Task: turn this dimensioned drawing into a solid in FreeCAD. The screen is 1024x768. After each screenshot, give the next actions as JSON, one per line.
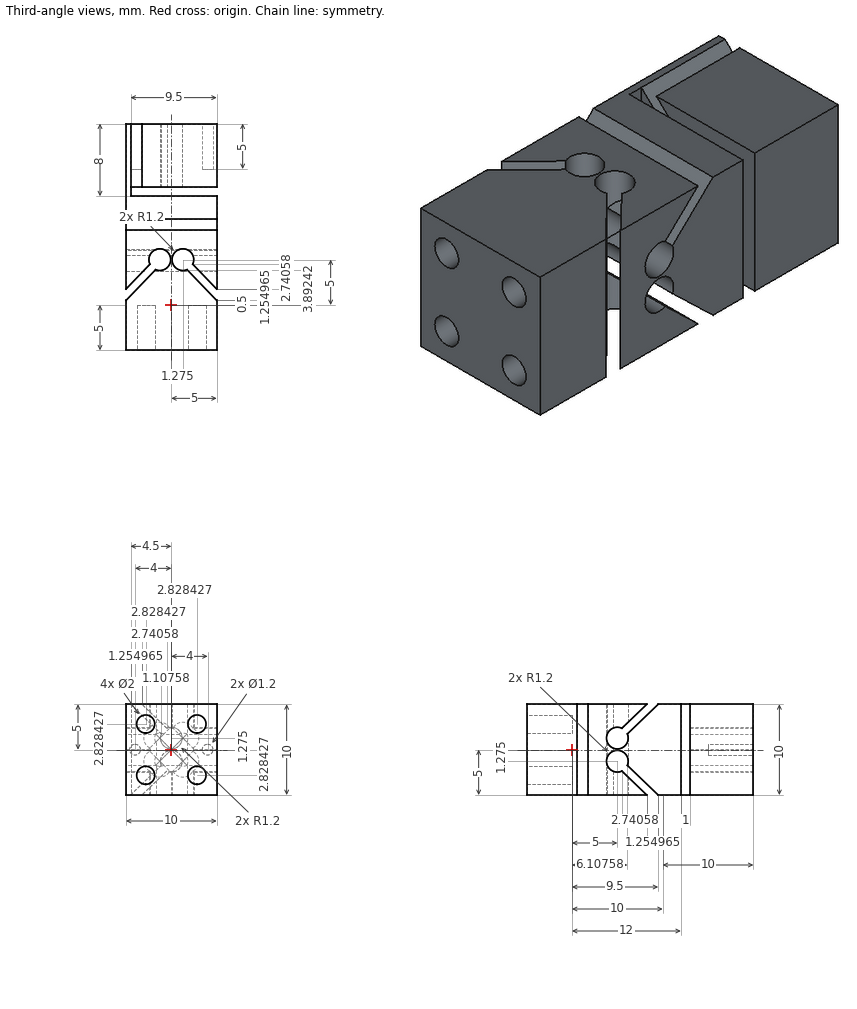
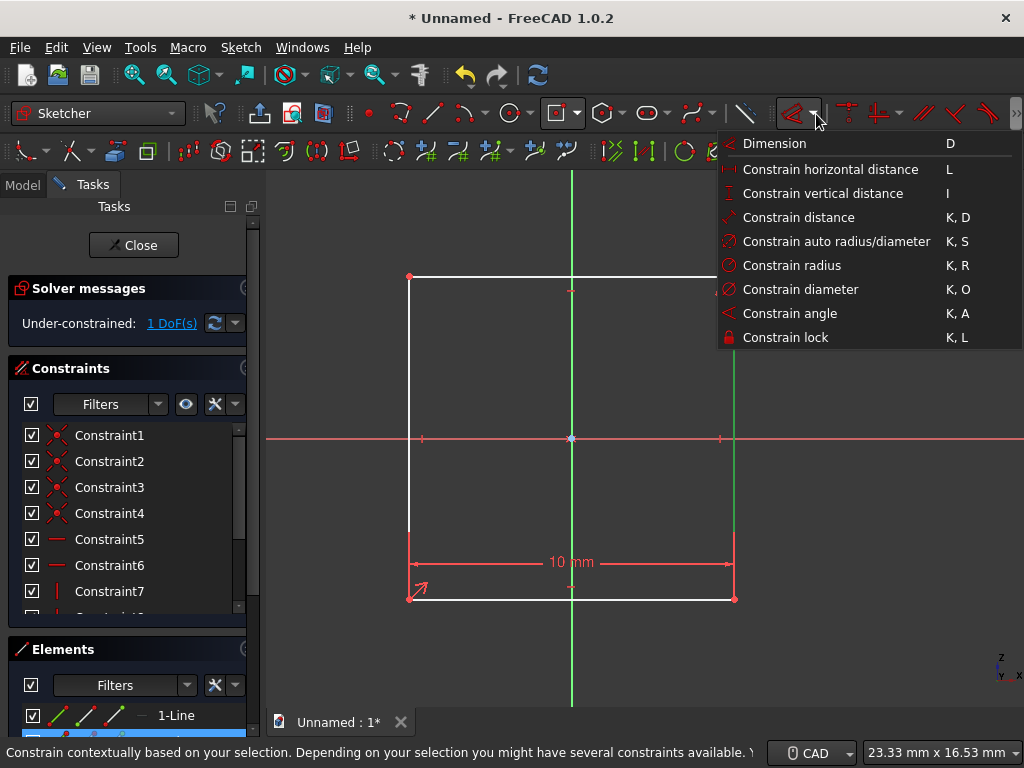
{"action": "left_click", "coordinate": [870, 193]}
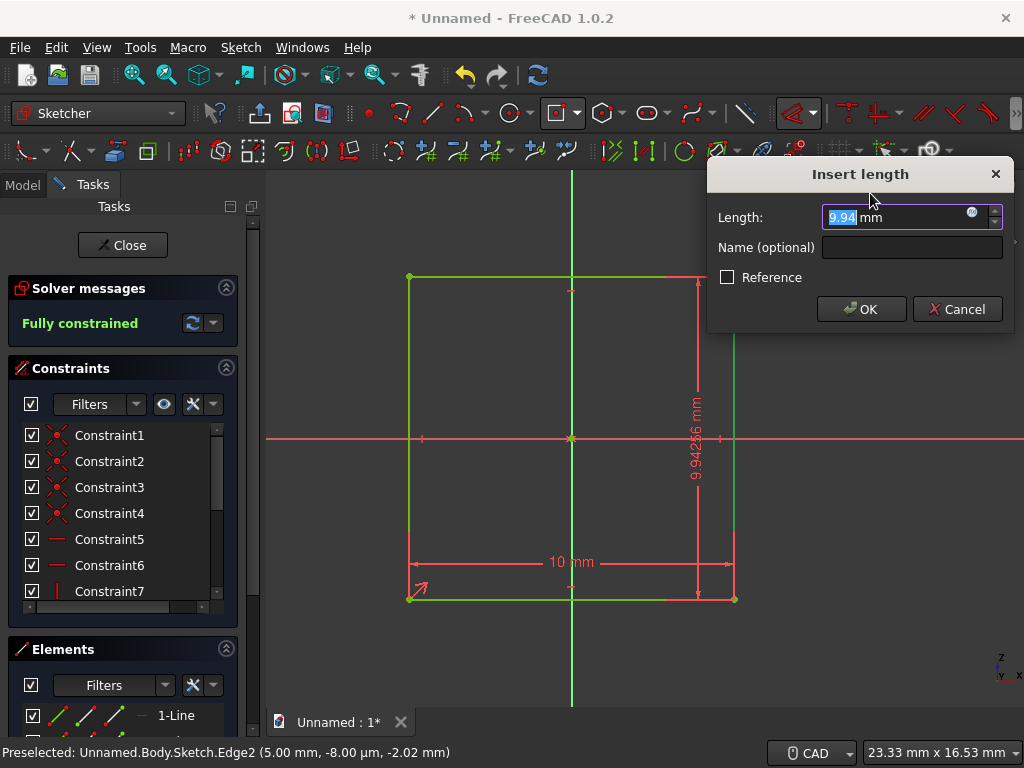
{"action": "type", "text": "10"}
{"action": "key", "text": "Return"}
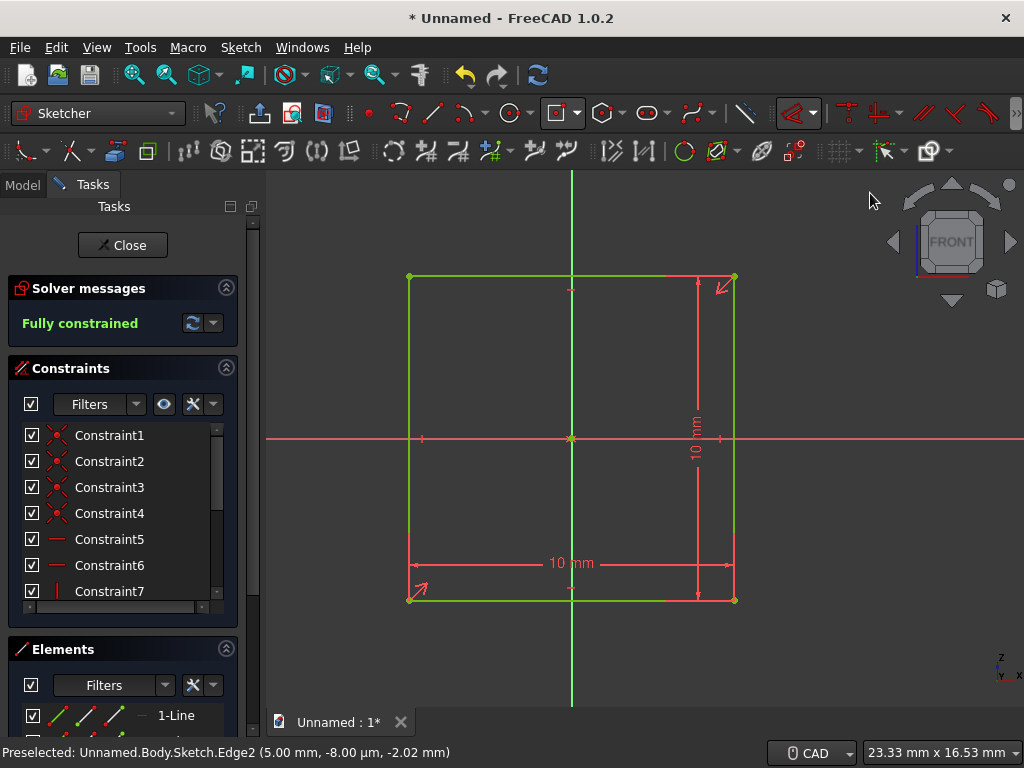
{"action": "left_click", "coordinate": [123, 245]}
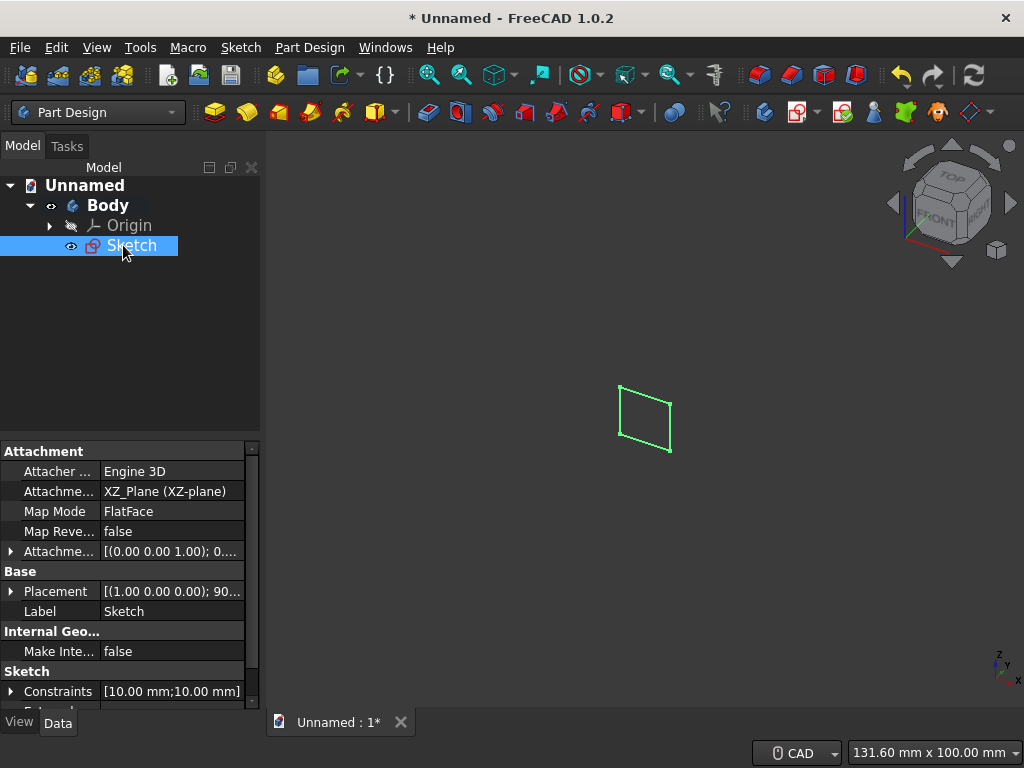
{"action": "left_click", "coordinate": [216, 112]}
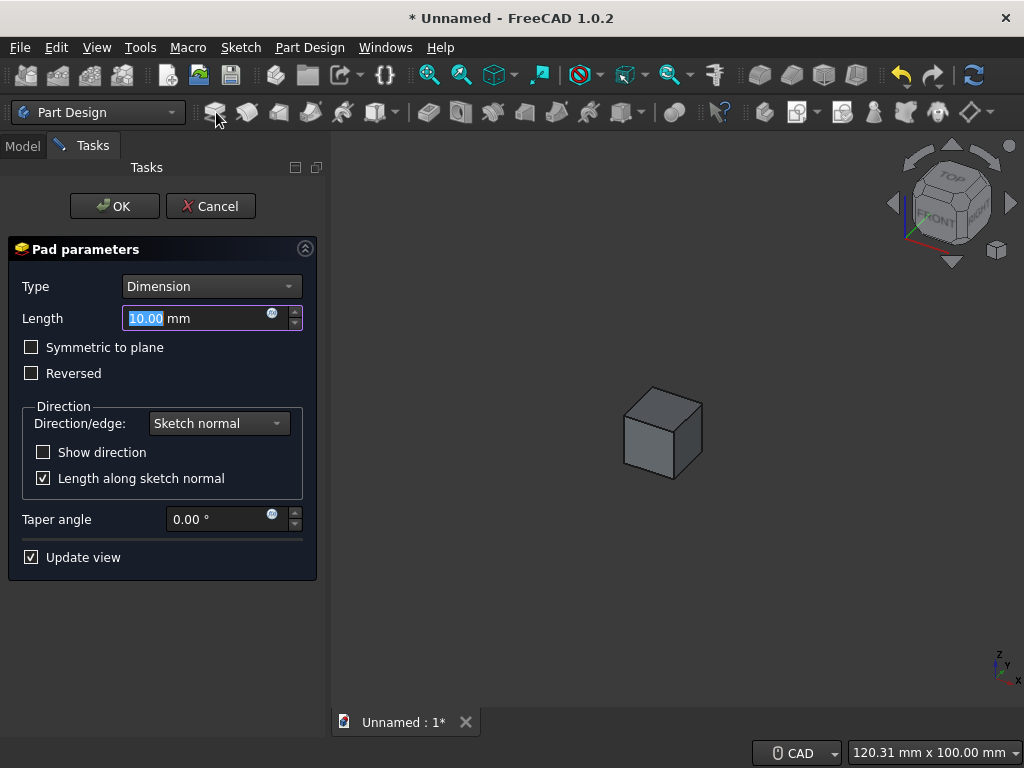
{"action": "type", "text": "10"}
{"action": "key", "text": "Tab"}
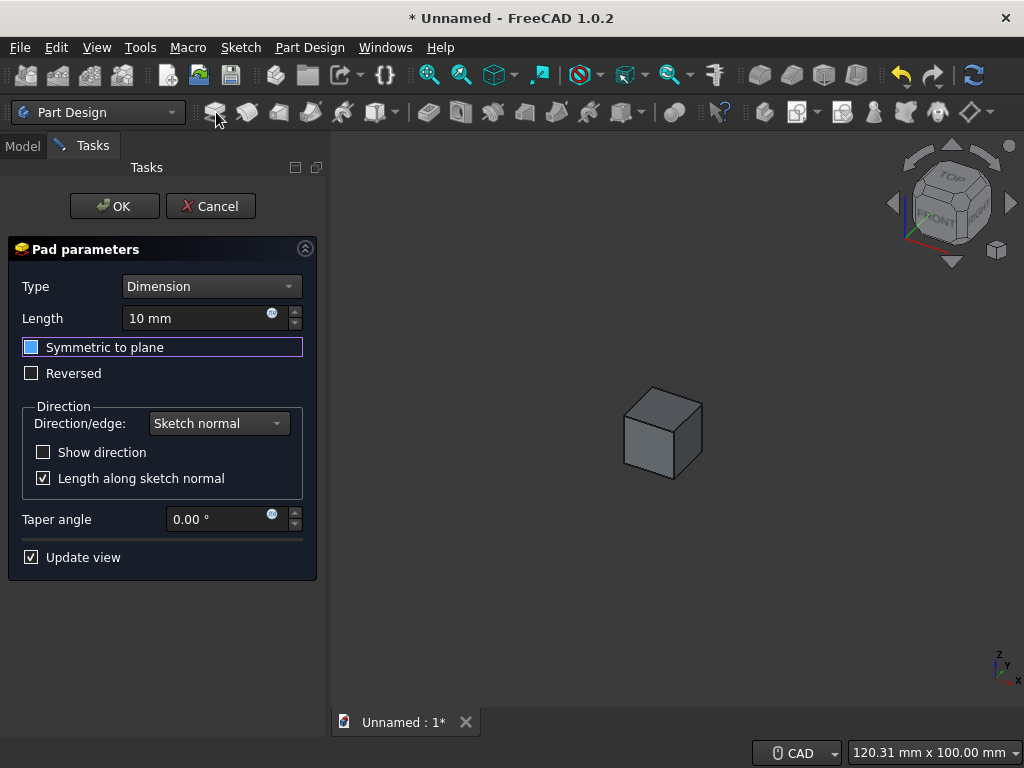
{"action": "left_click", "coordinate": [30, 373]}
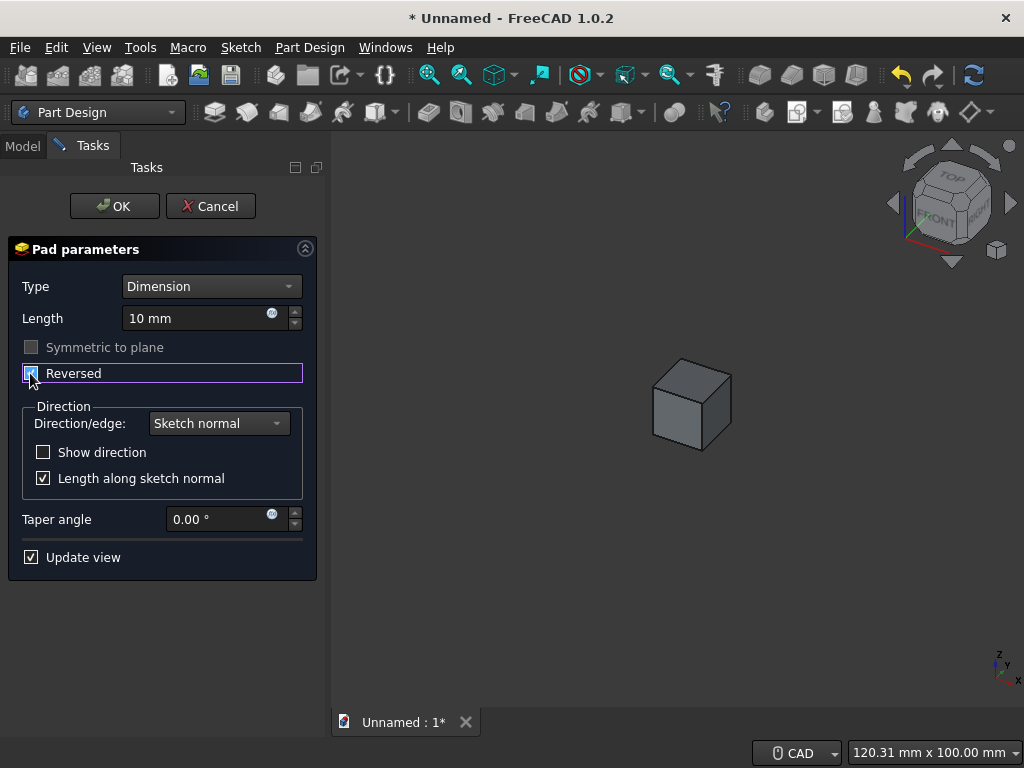
{"action": "left_click", "coordinate": [115, 206]}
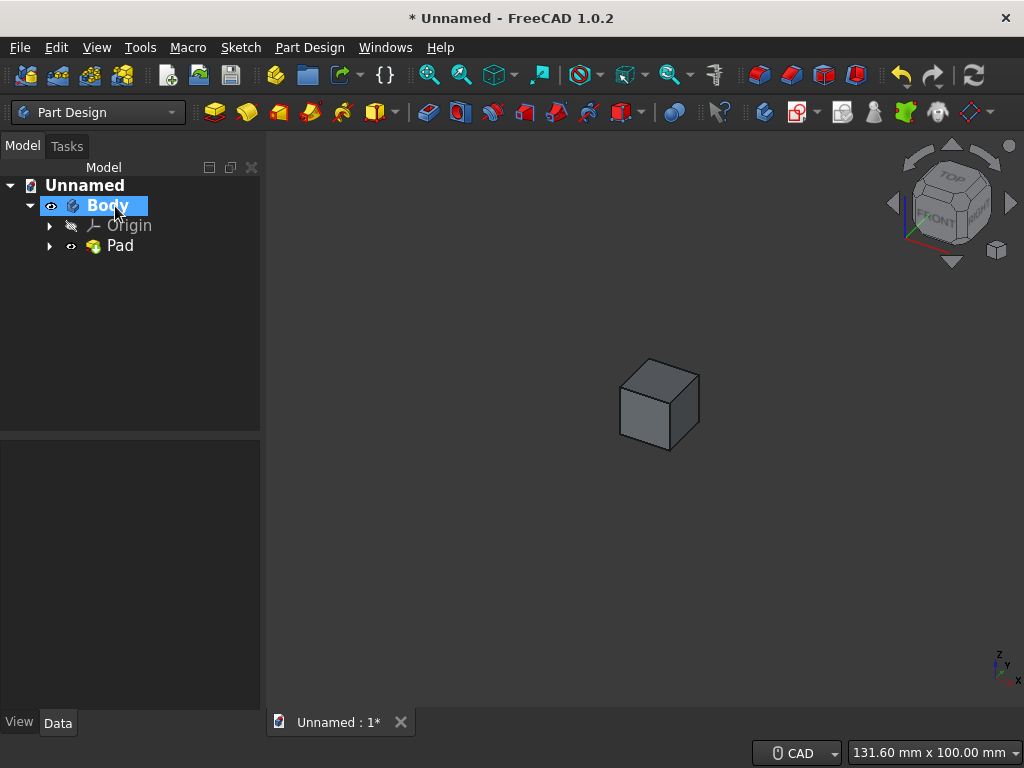
{"action": "key", "text": "v f"}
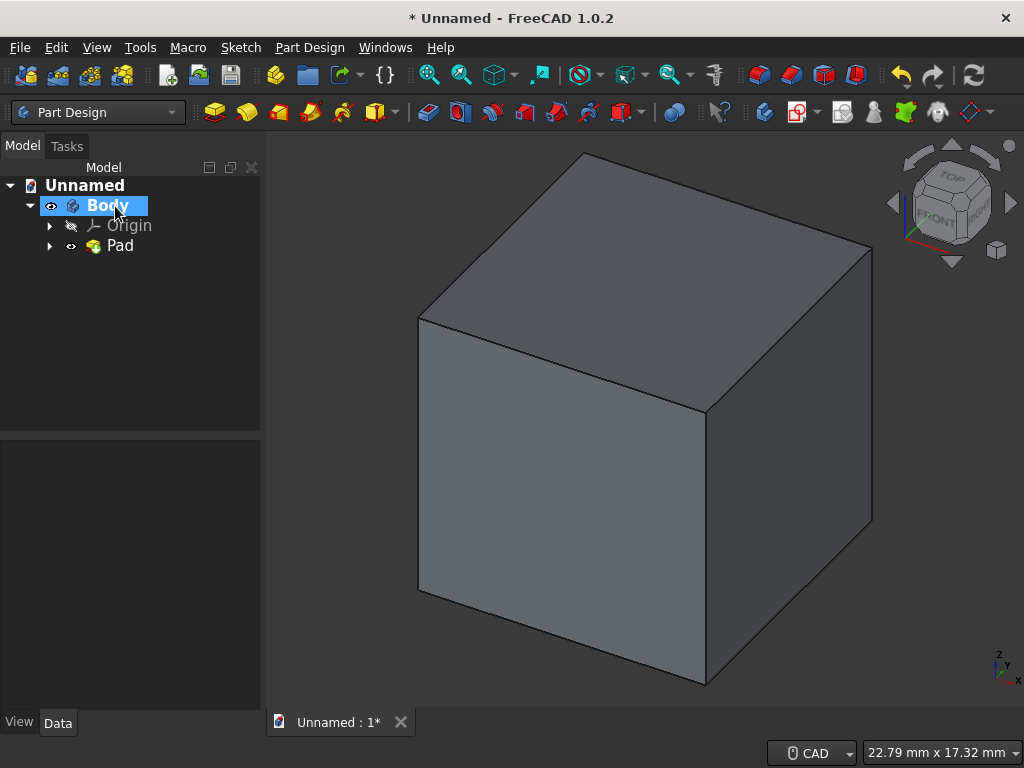
{"action": "left_click", "coordinate": [645, 282]}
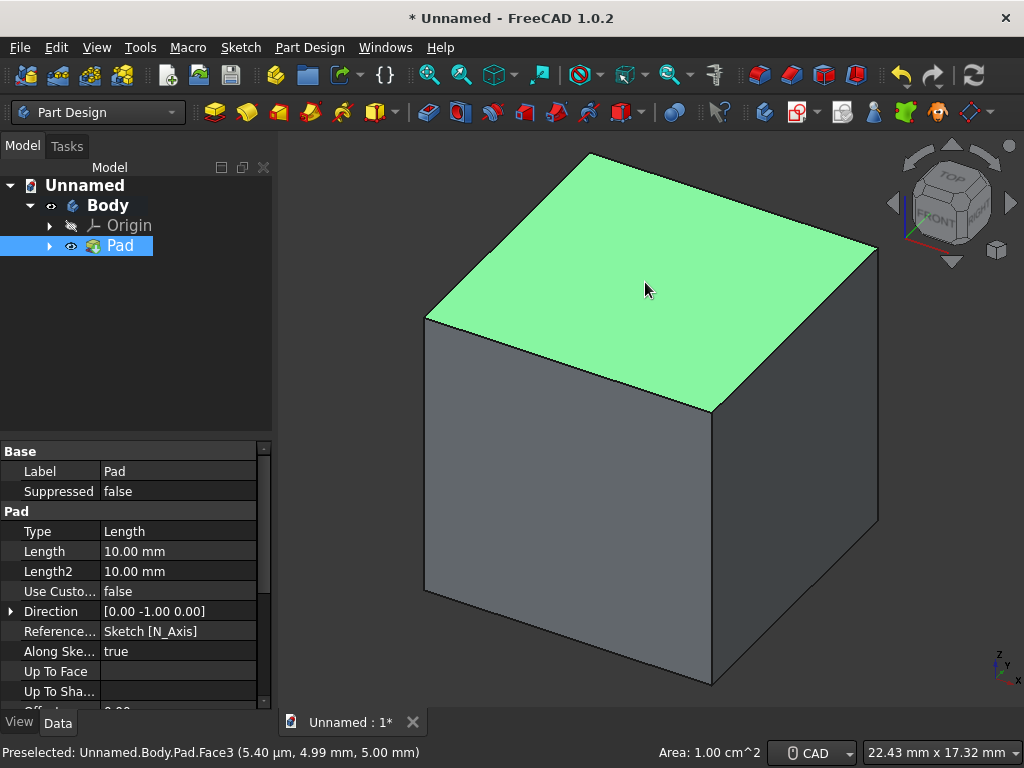
{"action": "left_click", "coordinate": [798, 112]}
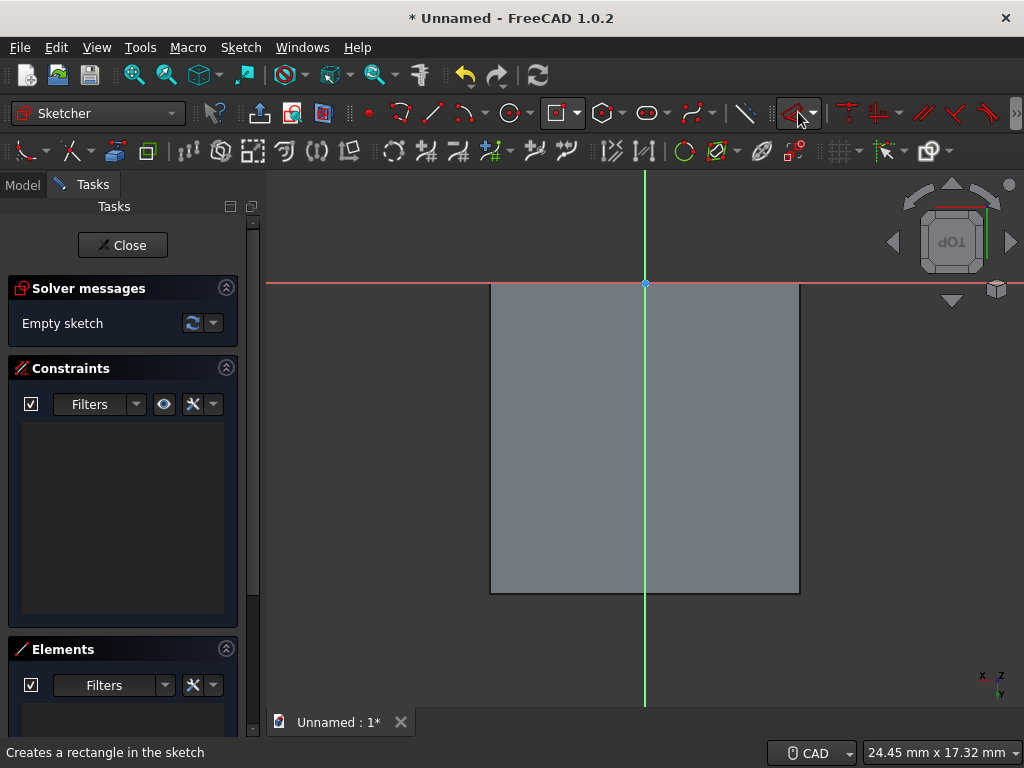
{"action": "left_click", "coordinate": [402, 114]}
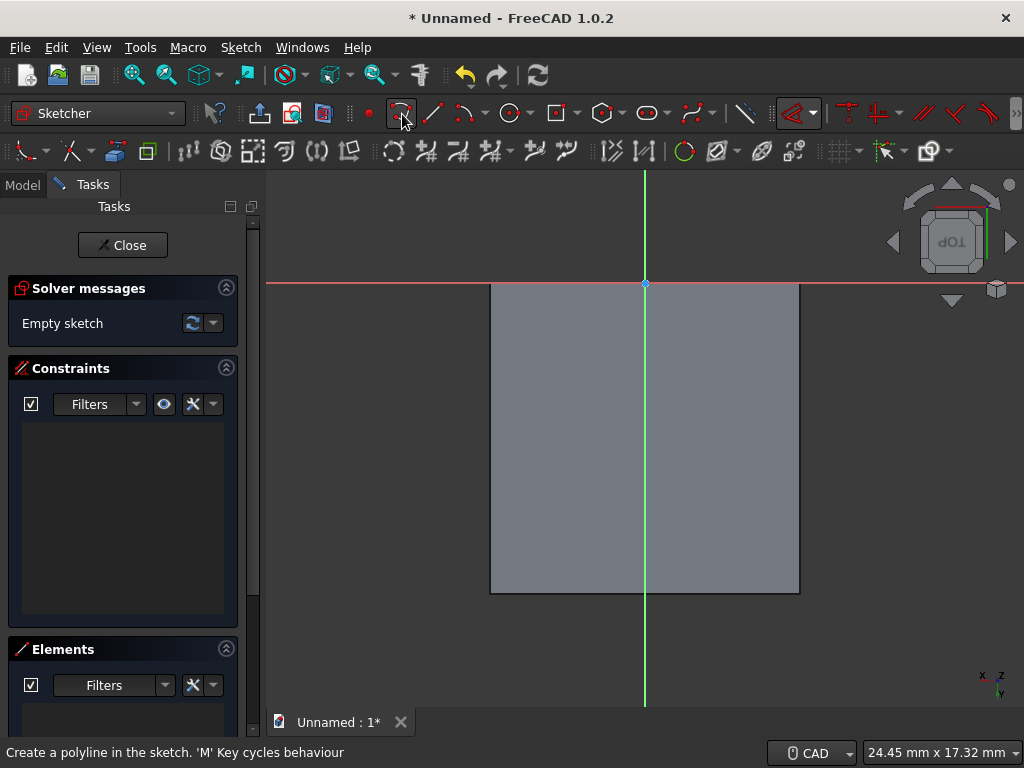
{"action": "left_click", "coordinate": [591, 404]}
{"action": "left_click", "coordinate": [490, 299]}
{"action": "left_click", "coordinate": [490, 338]}
{"action": "left_click", "coordinate": [572, 423]}
{"action": "right_click", "coordinate": [572, 423]}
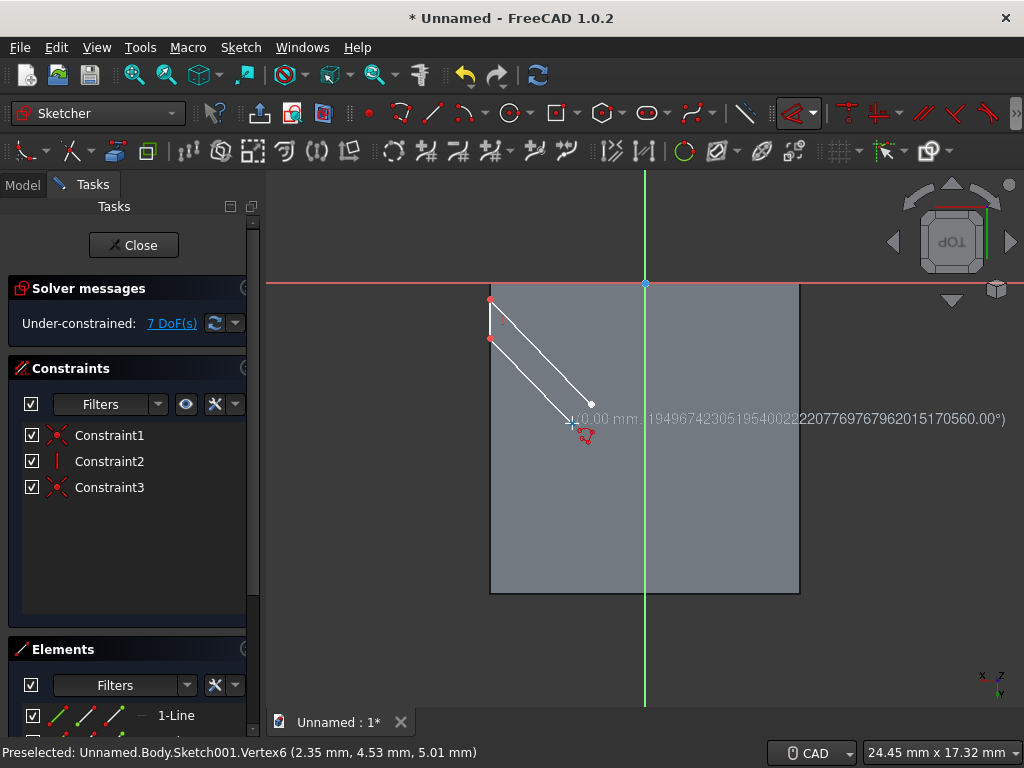
{"action": "key", "text": "g 3 a"}